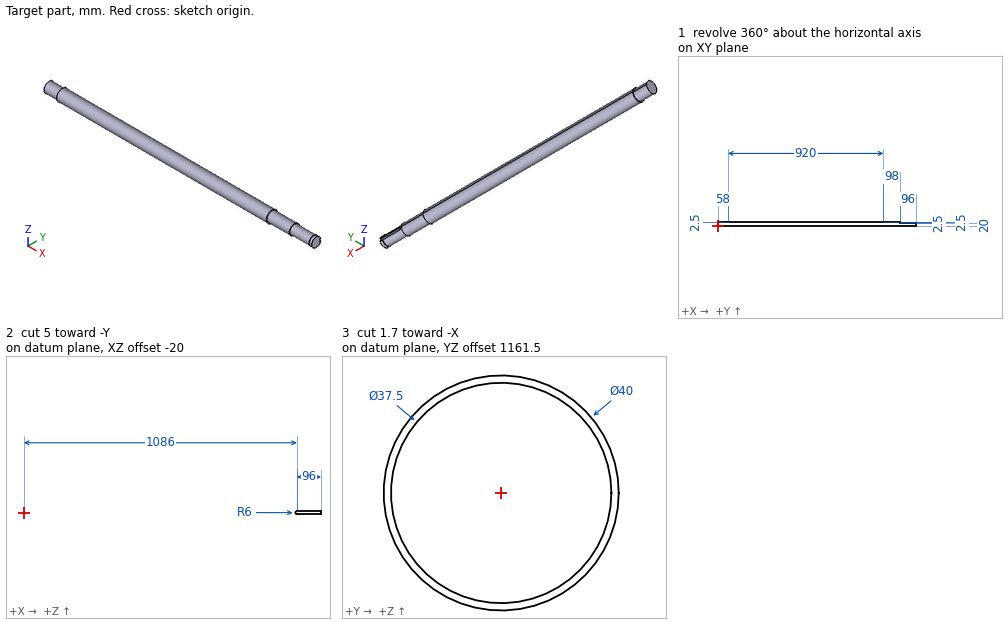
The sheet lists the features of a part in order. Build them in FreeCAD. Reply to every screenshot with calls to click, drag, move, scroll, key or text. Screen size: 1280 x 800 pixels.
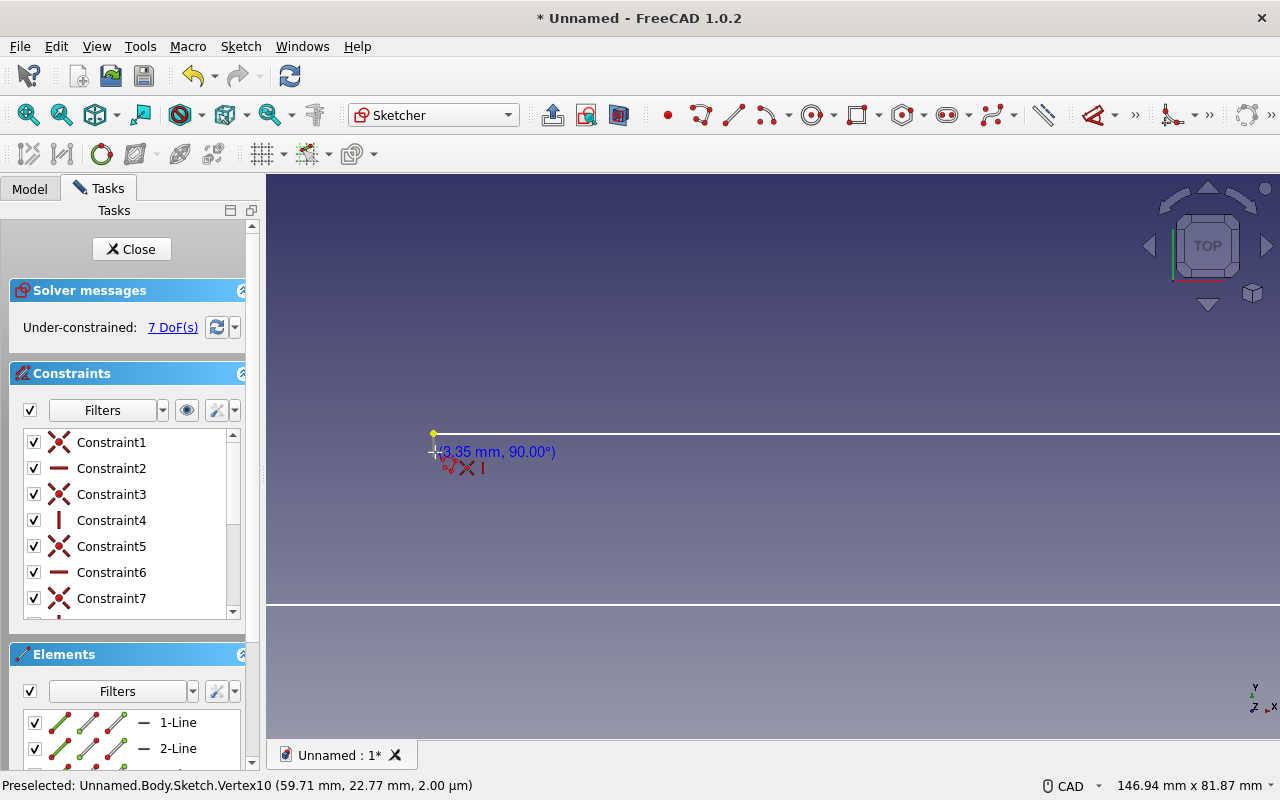
click(434, 450)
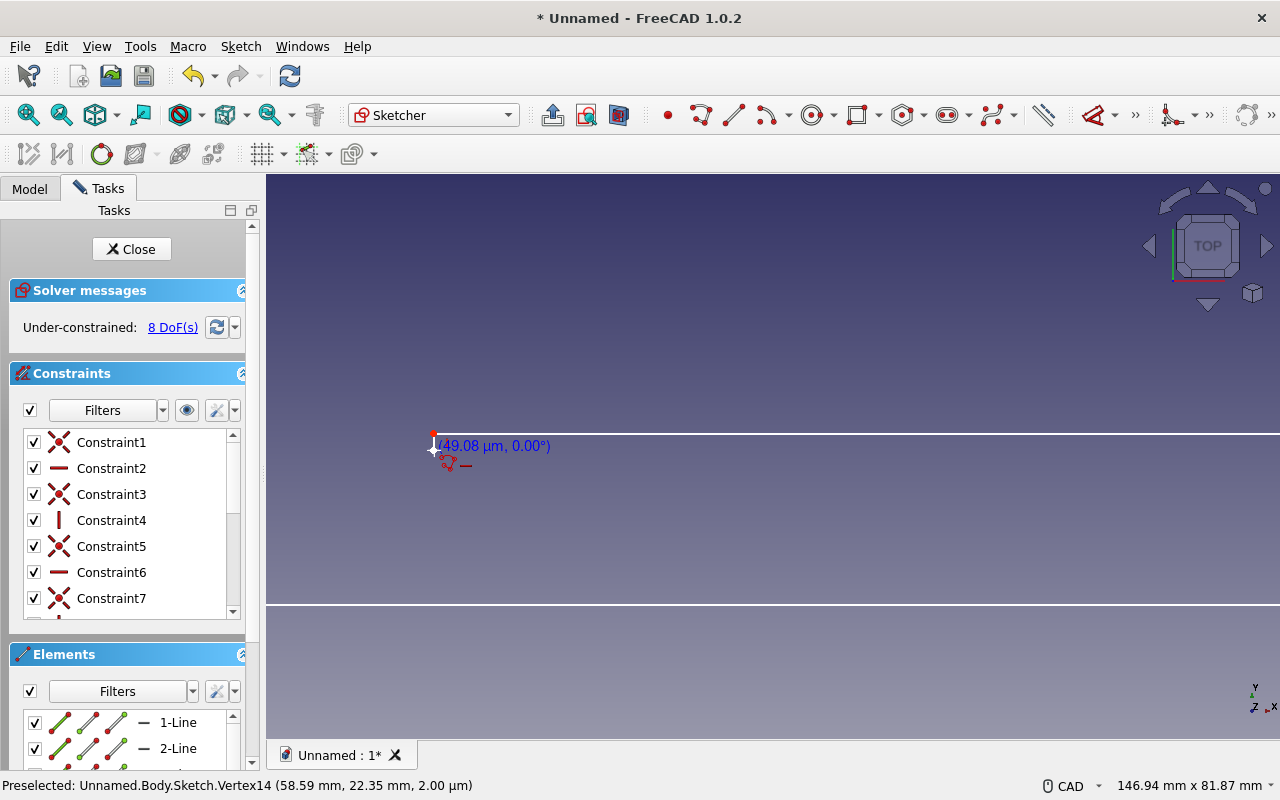
scroll(434, 451, down, 13)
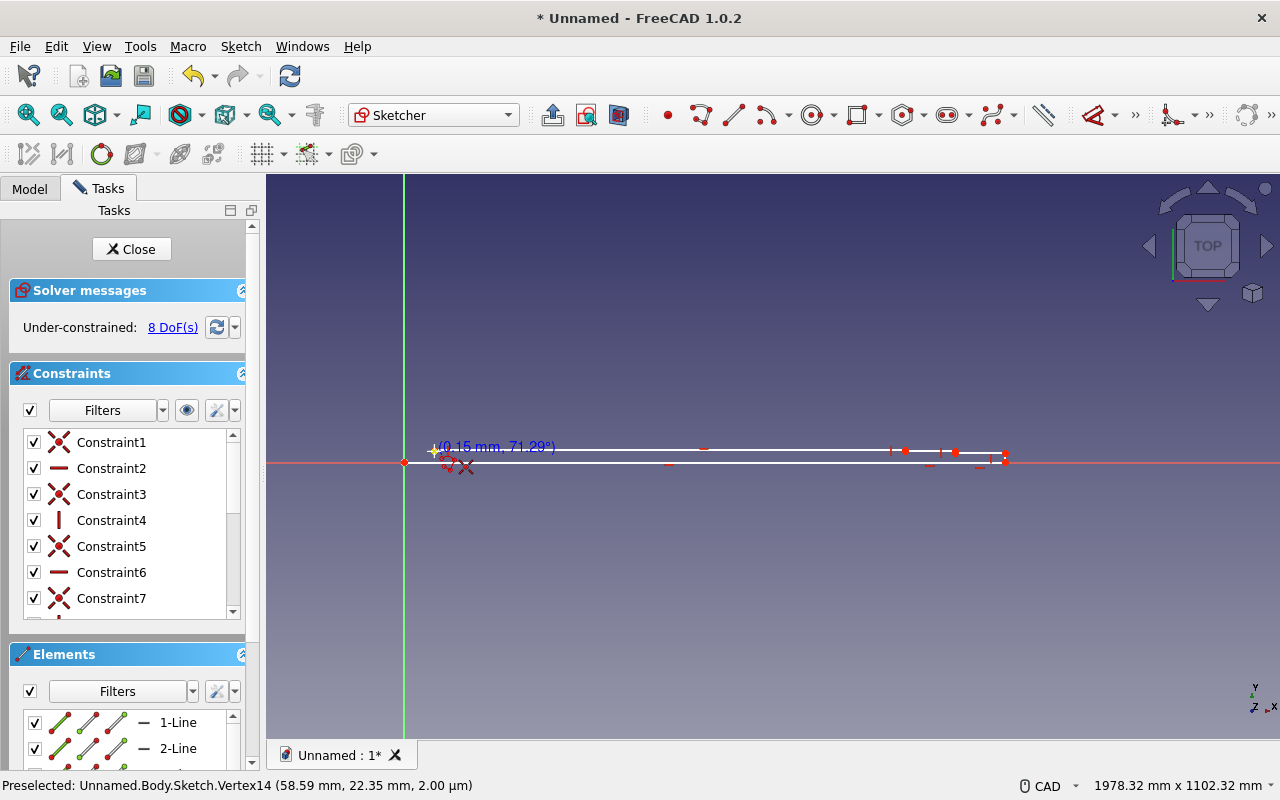
scroll(404, 451, up, 2)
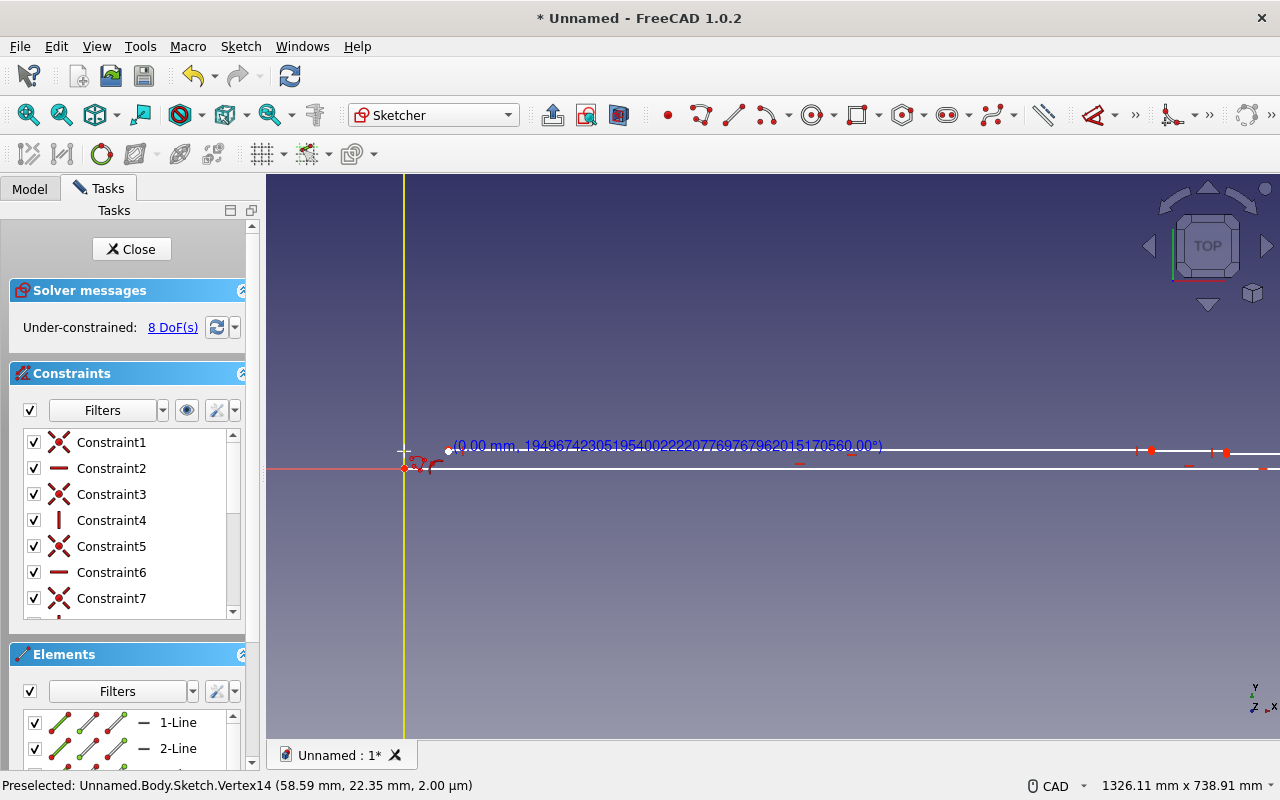
click(413, 451)
click(404, 469)
key(Escape)
key(Escape)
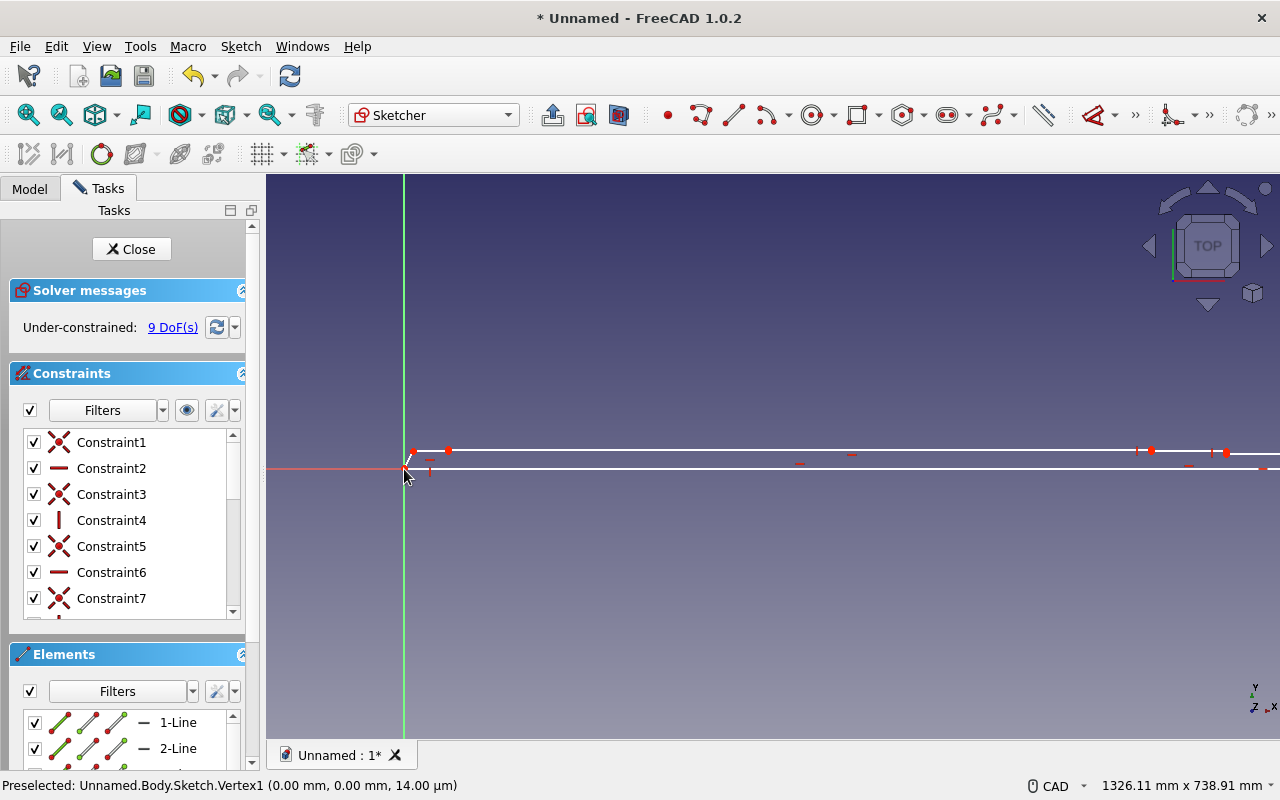
scroll(408, 462, up, 4)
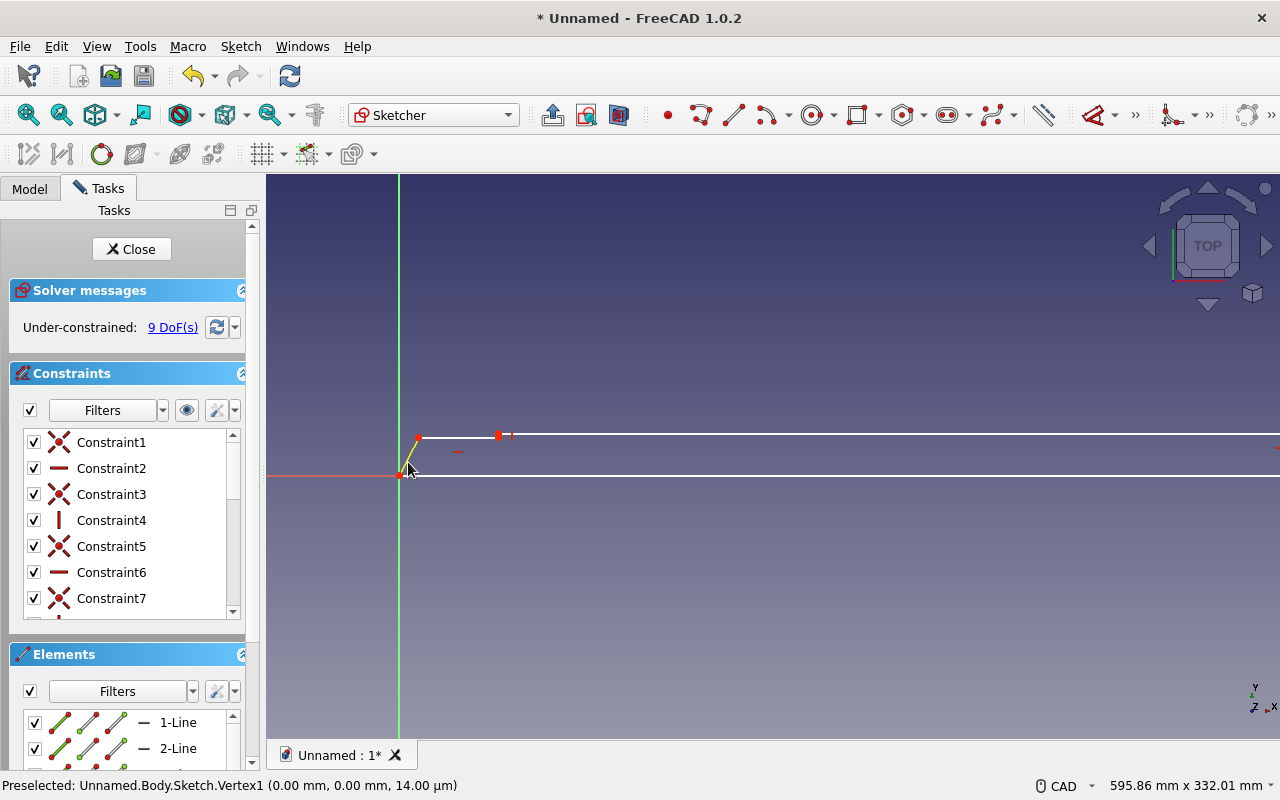
click(407, 461)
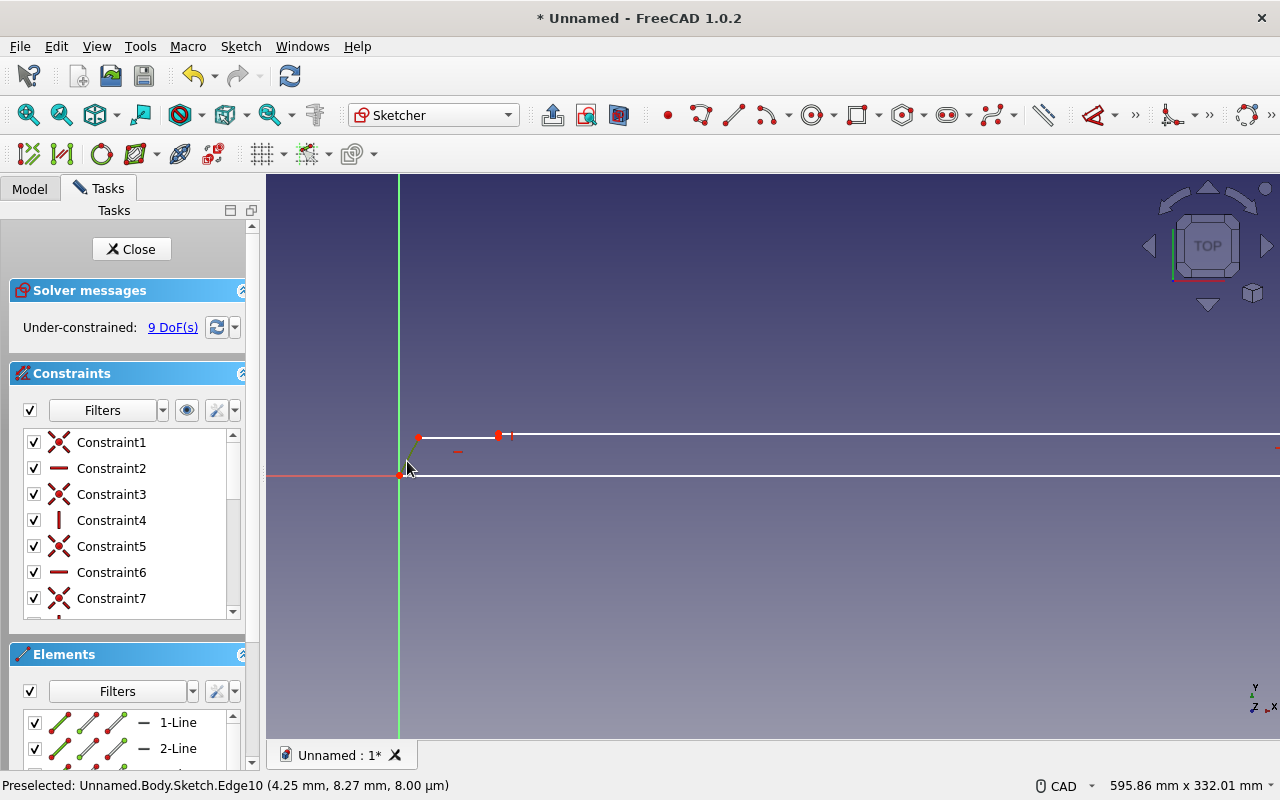
key(v)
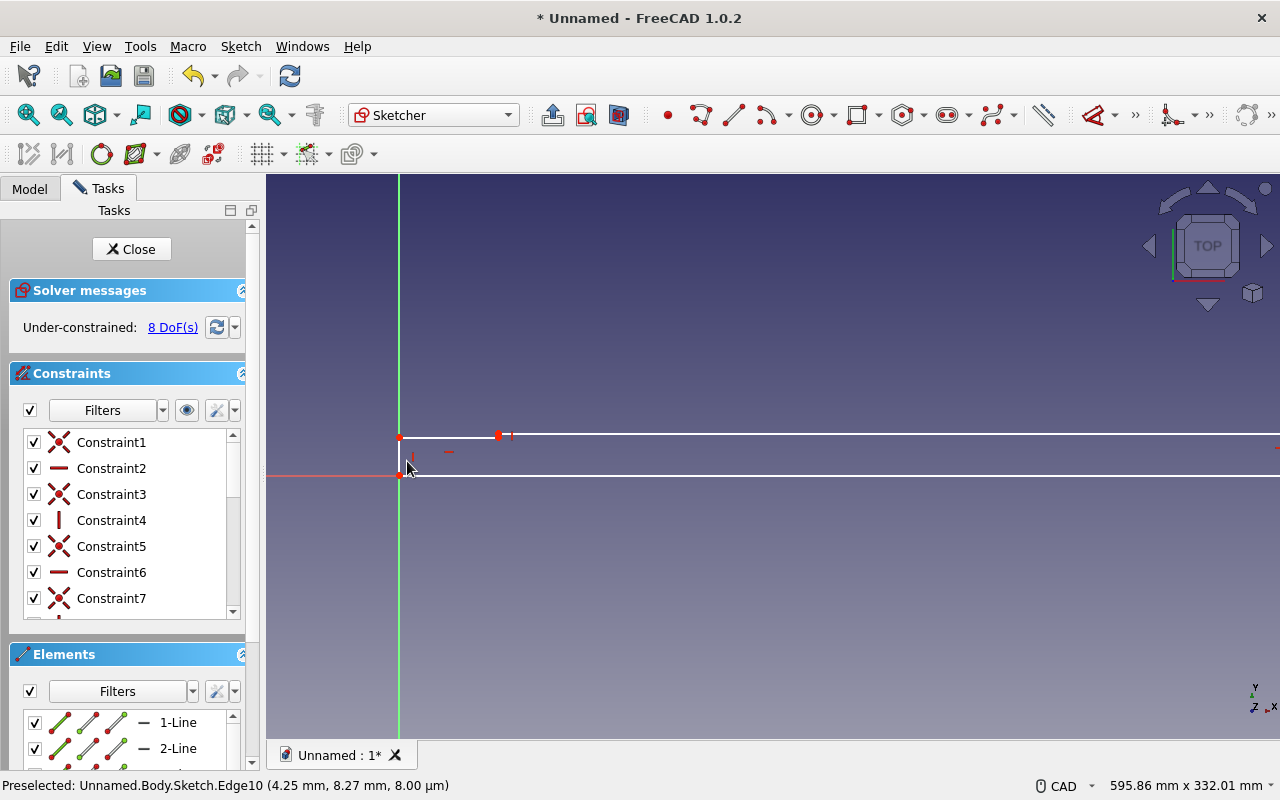
click(1092, 116)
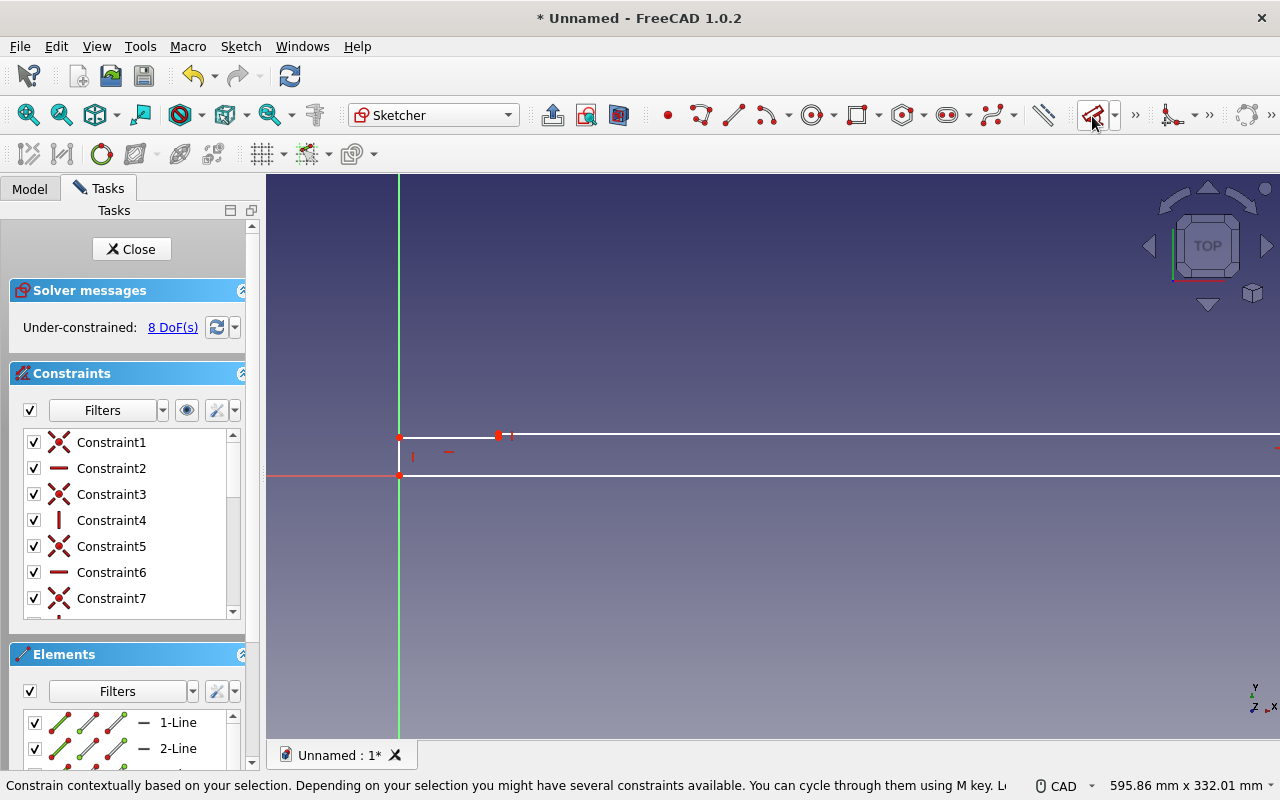
scroll(406, 457, down, 6)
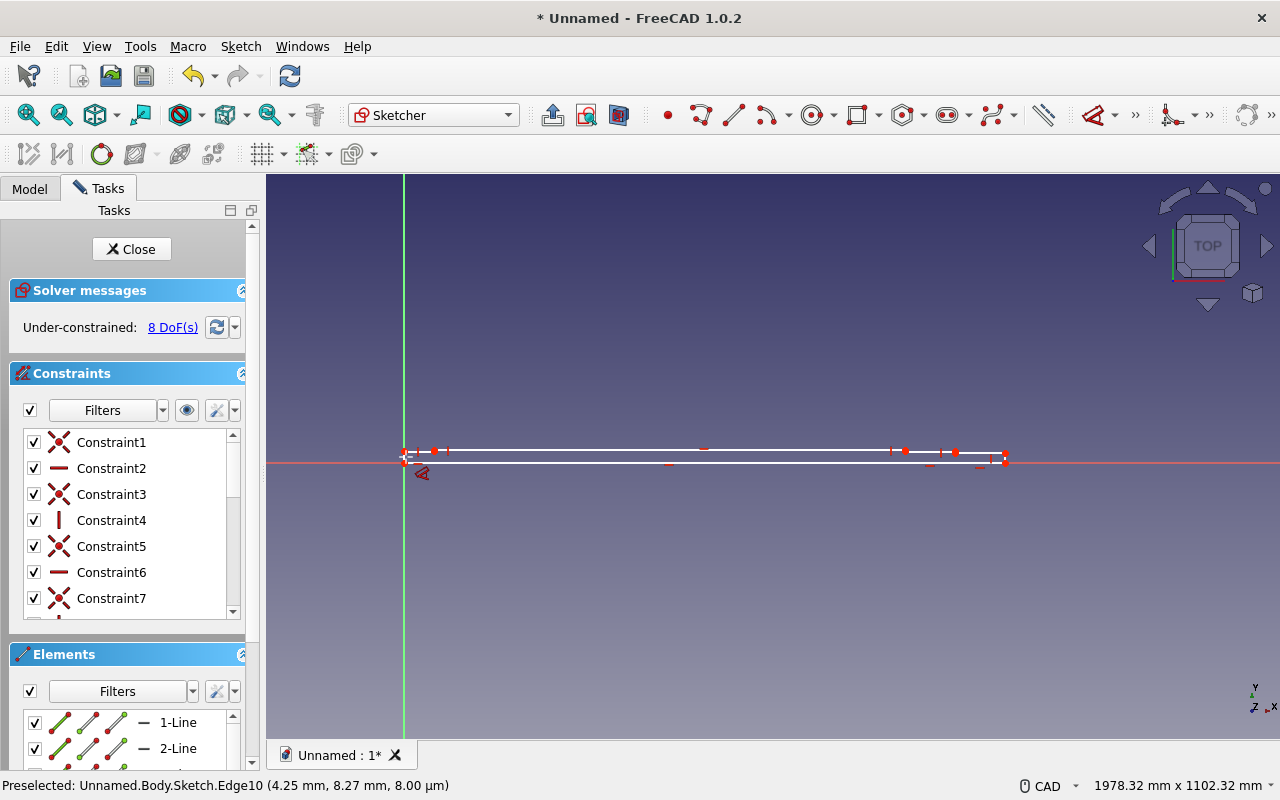
scroll(1005, 460, up, 8)